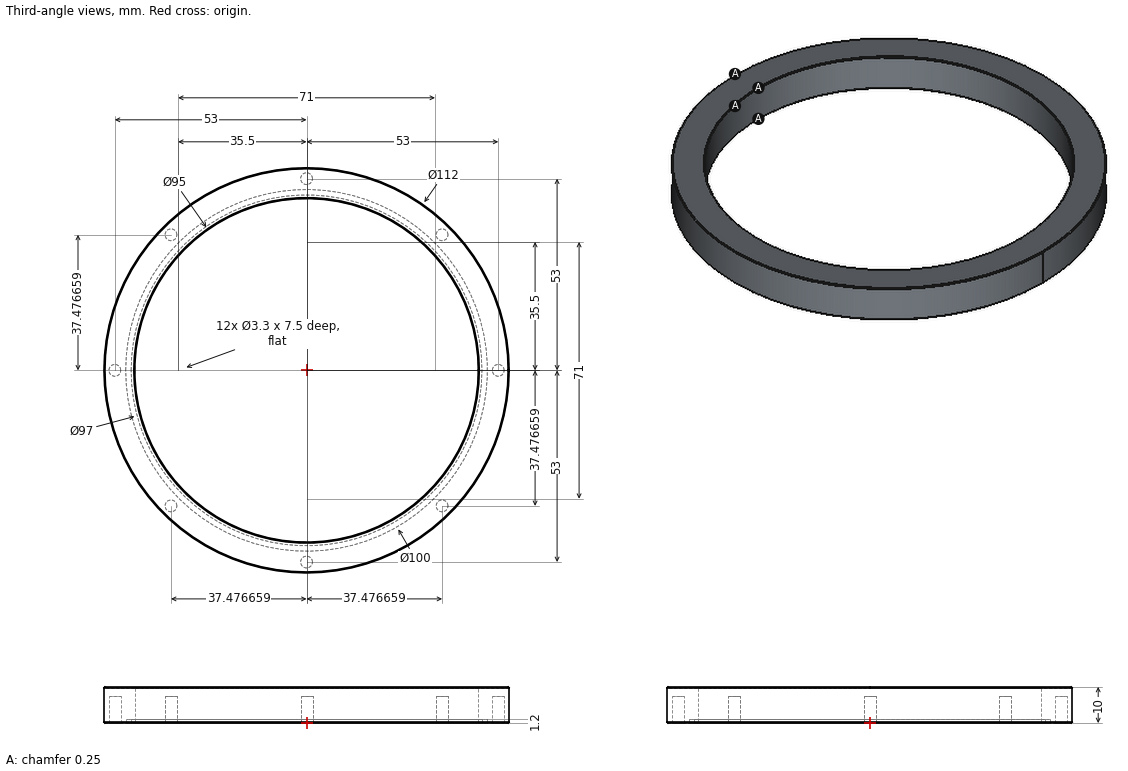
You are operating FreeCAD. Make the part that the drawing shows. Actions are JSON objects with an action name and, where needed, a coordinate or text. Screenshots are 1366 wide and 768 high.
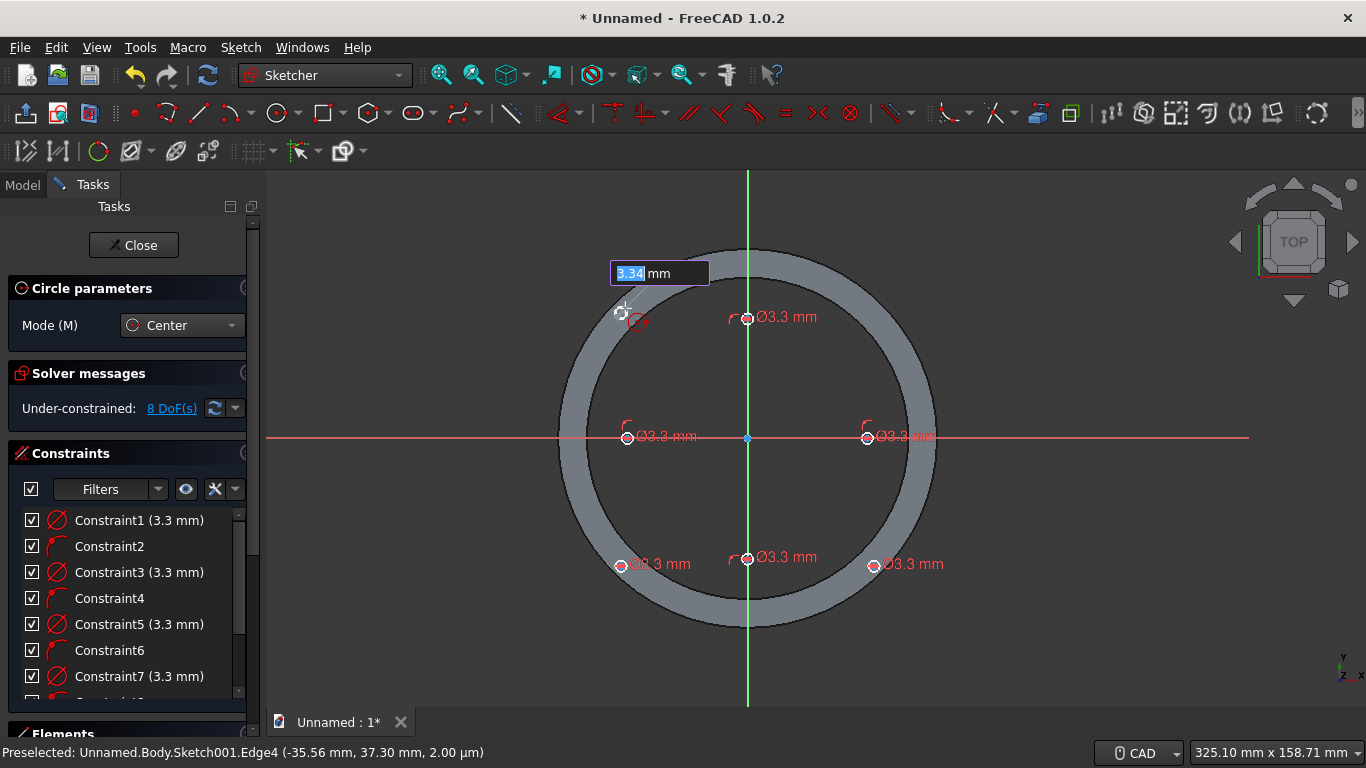
{"action": "type", "text": "3.3"}
{"action": "key", "text": "Return"}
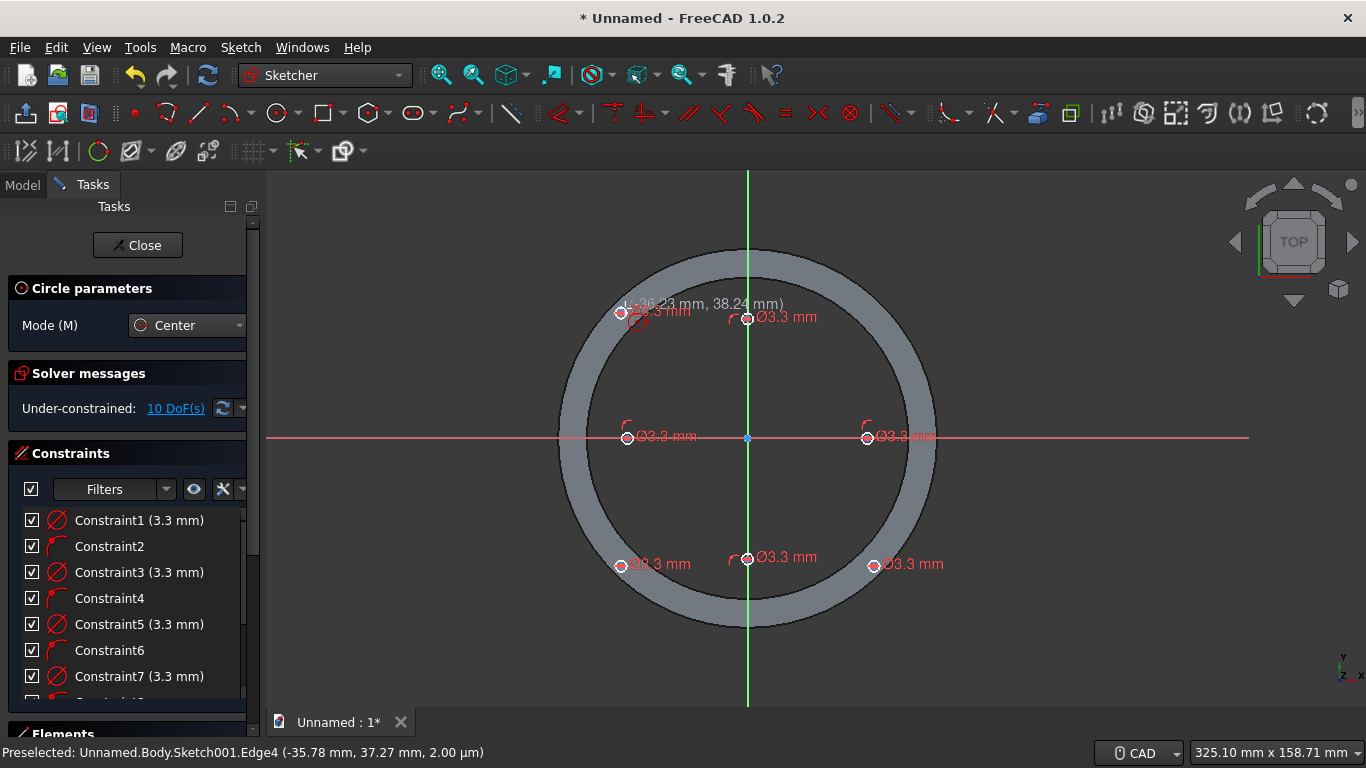
{"action": "scroll", "coordinate": [874, 312], "scroll_direction": "up", "scroll_amount": 8}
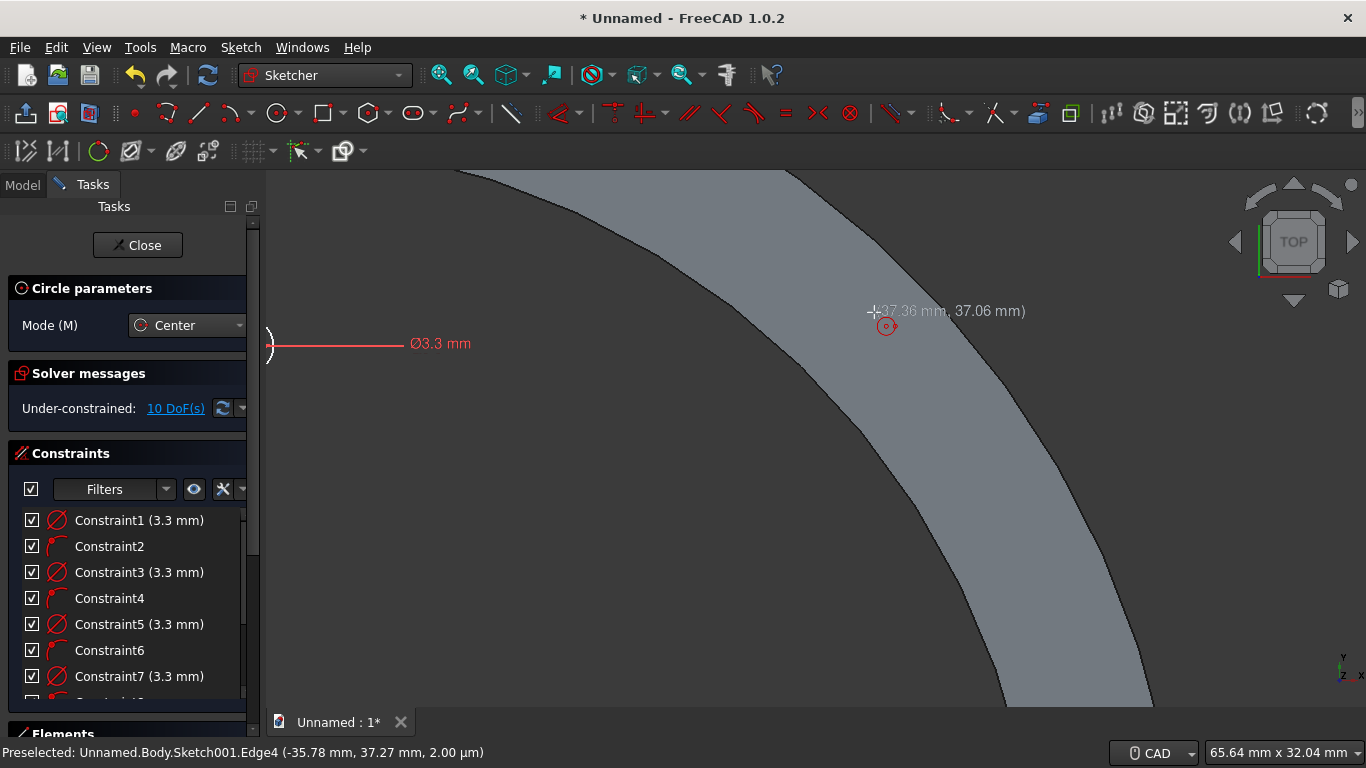
{"action": "scroll", "coordinate": [874, 312], "scroll_direction": "down", "scroll_amount": 8}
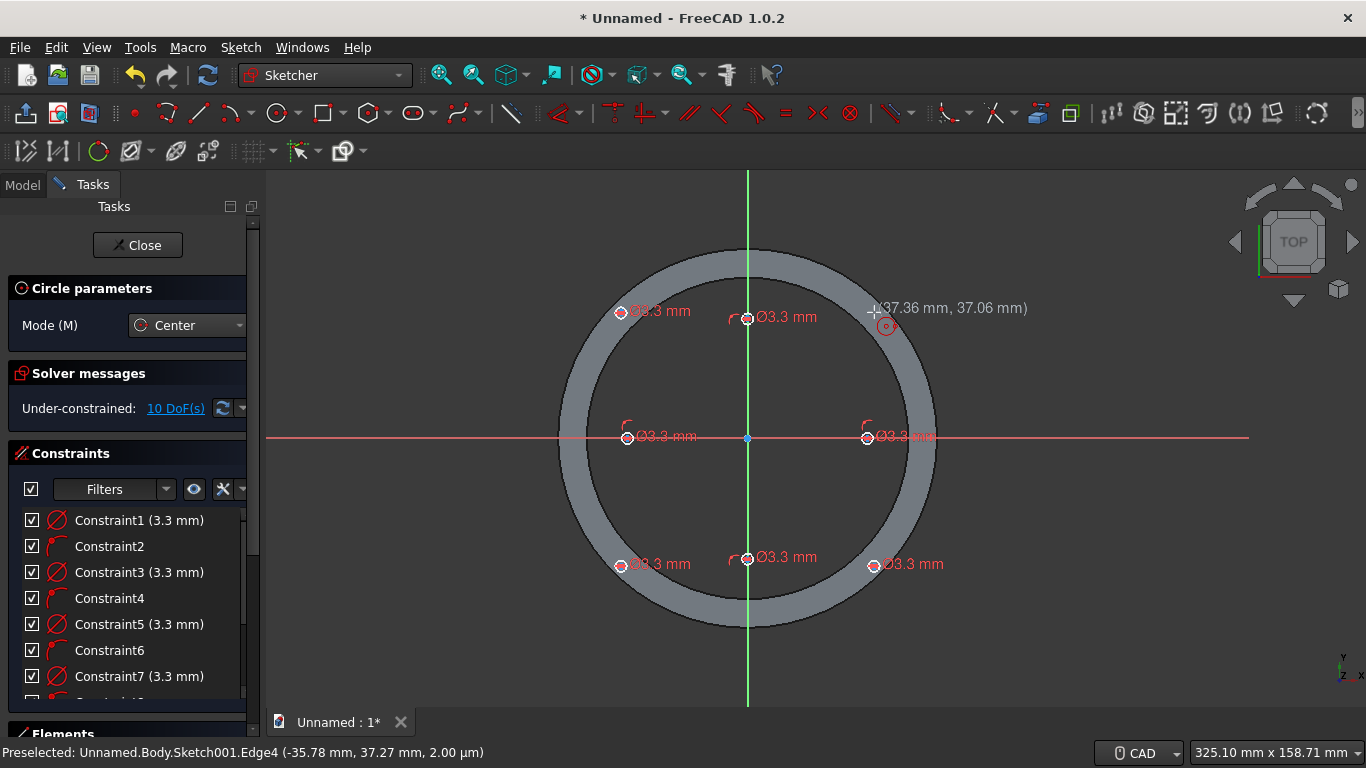
{"action": "left_click", "coordinate": [874, 312]}
{"action": "mouse_move", "coordinate": [878, 308]}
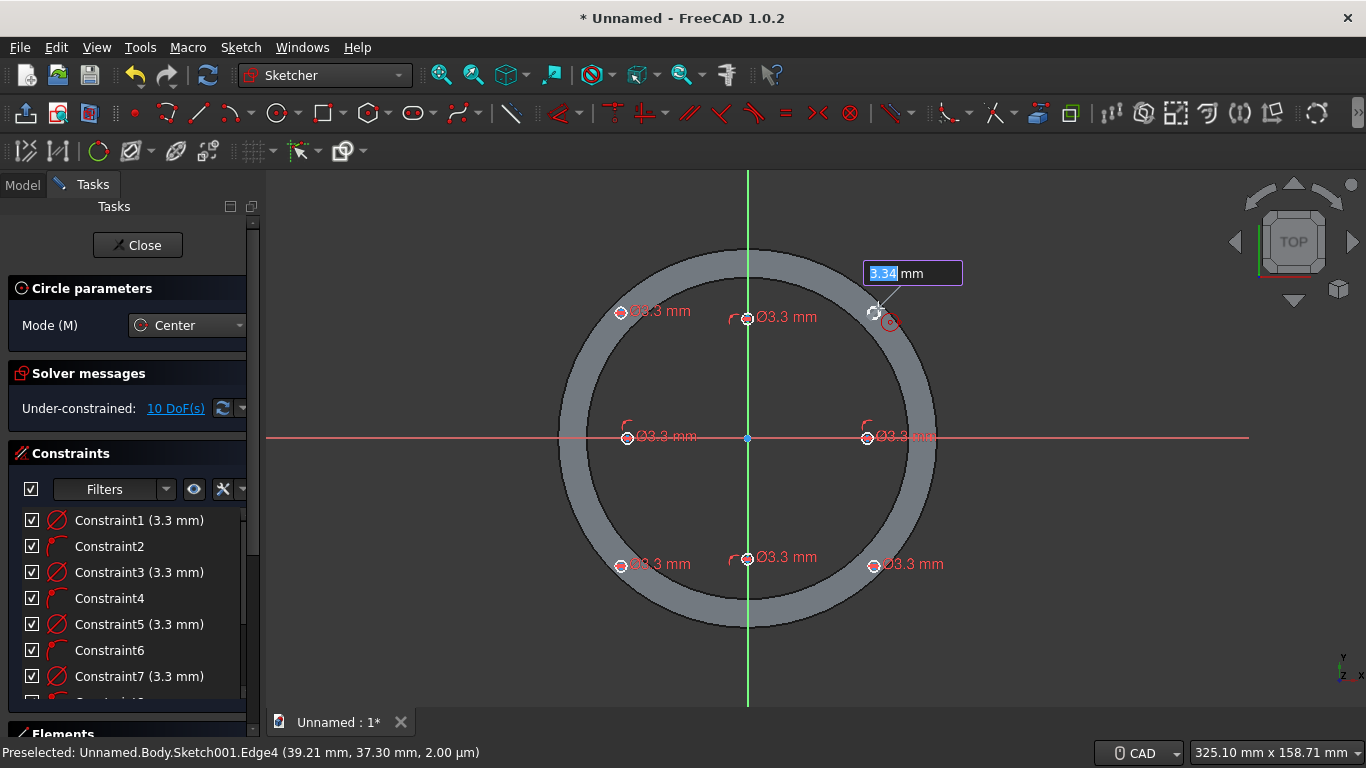
{"action": "type", "text": "3.3"}
{"action": "key", "text": "Return"}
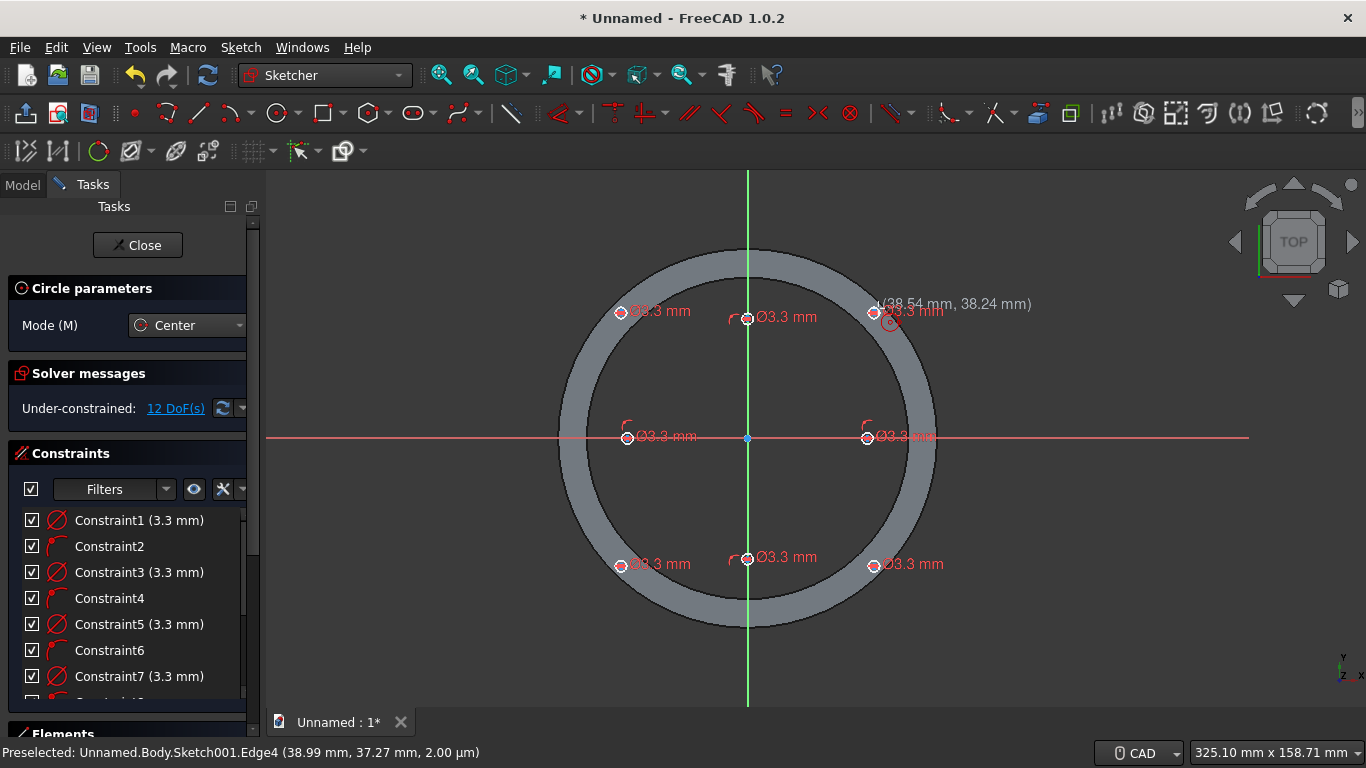
{"action": "scroll", "coordinate": [748, 259], "scroll_direction": "up", "scroll_amount": 8}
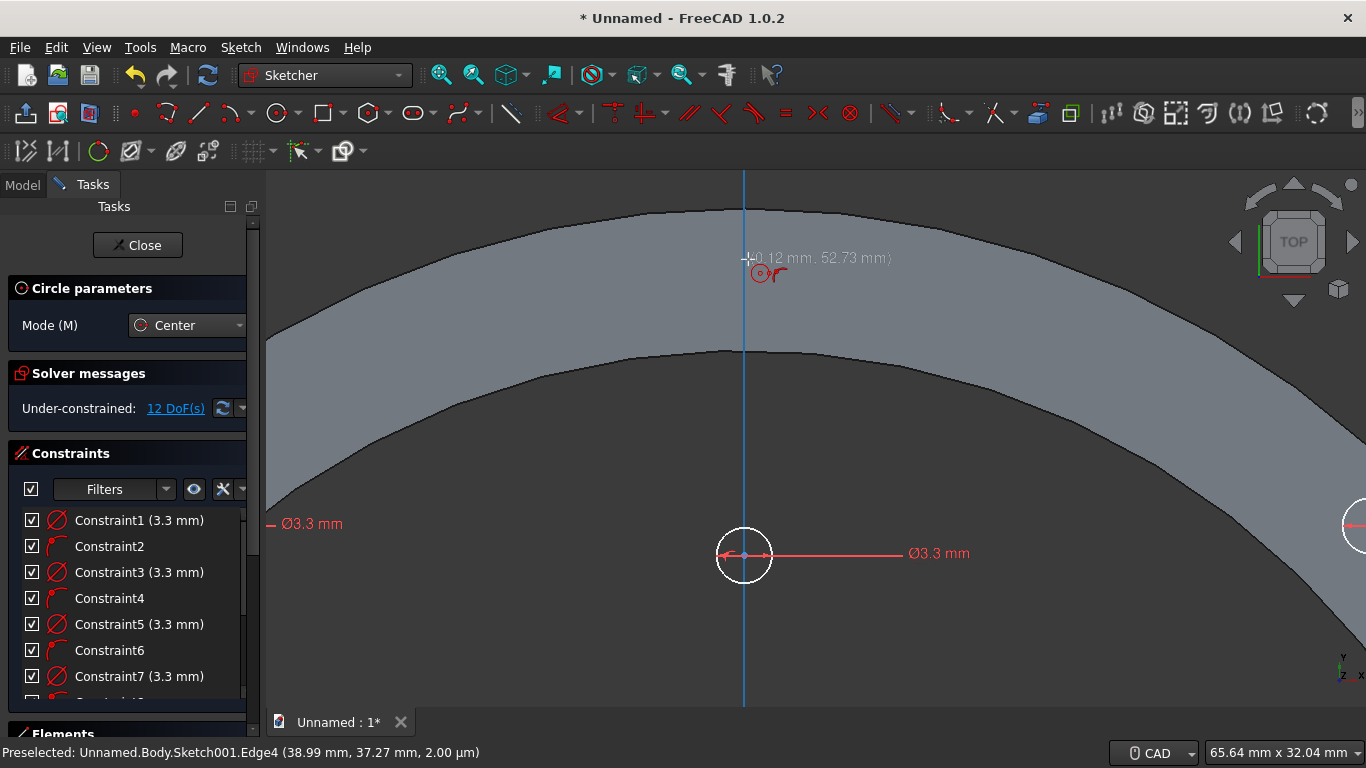
{"action": "scroll", "coordinate": [748, 259], "scroll_direction": "down", "scroll_amount": 8}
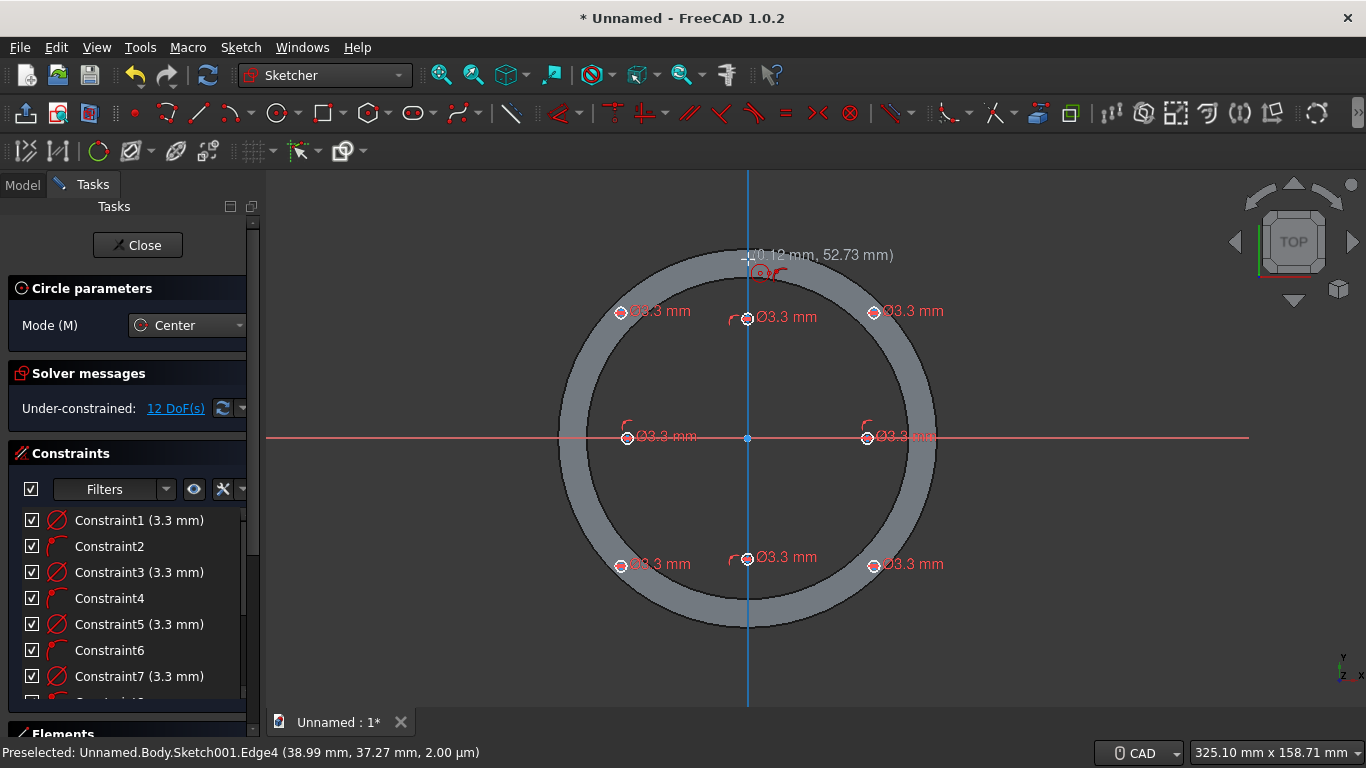
{"action": "left_click", "coordinate": [748, 259]}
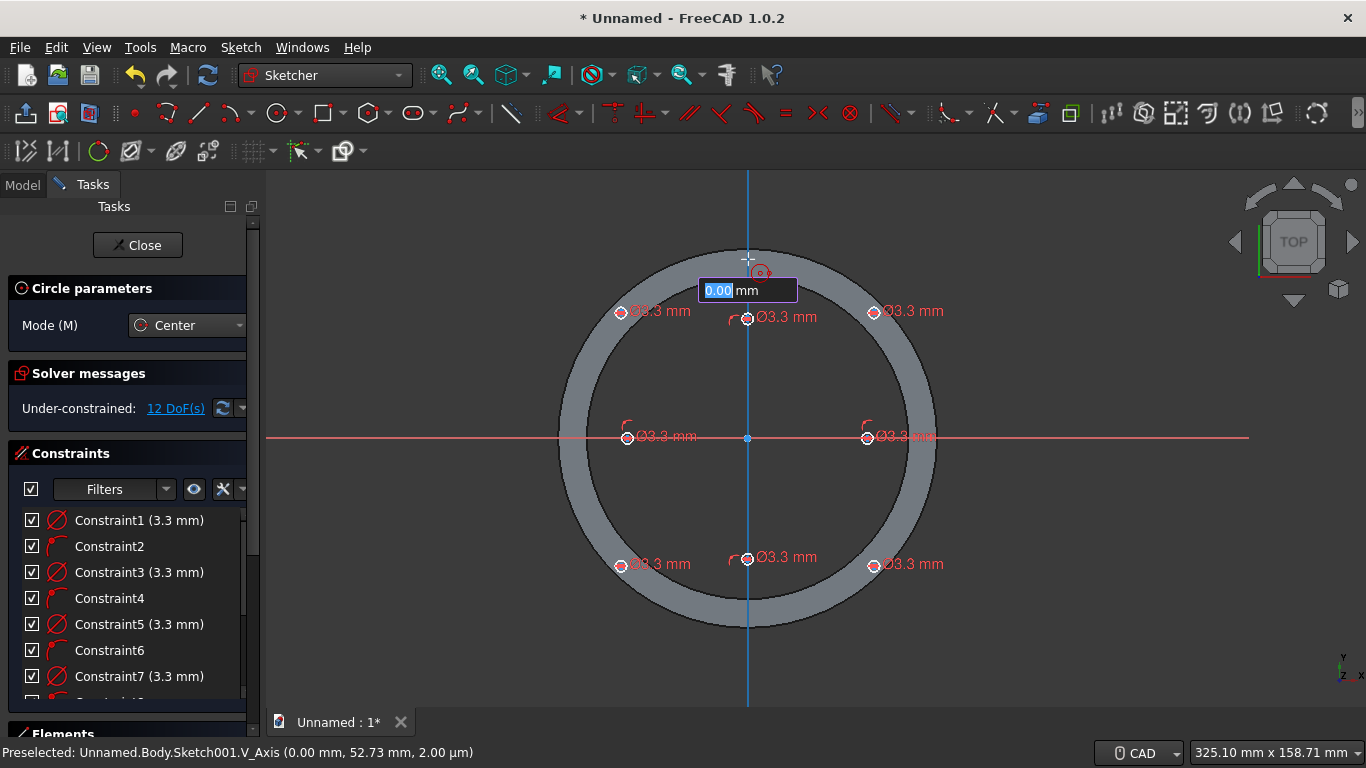
{"action": "scroll", "coordinate": [753, 257], "scroll_direction": "up", "scroll_amount": 6}
{"action": "mouse_move", "coordinate": [751, 257]}